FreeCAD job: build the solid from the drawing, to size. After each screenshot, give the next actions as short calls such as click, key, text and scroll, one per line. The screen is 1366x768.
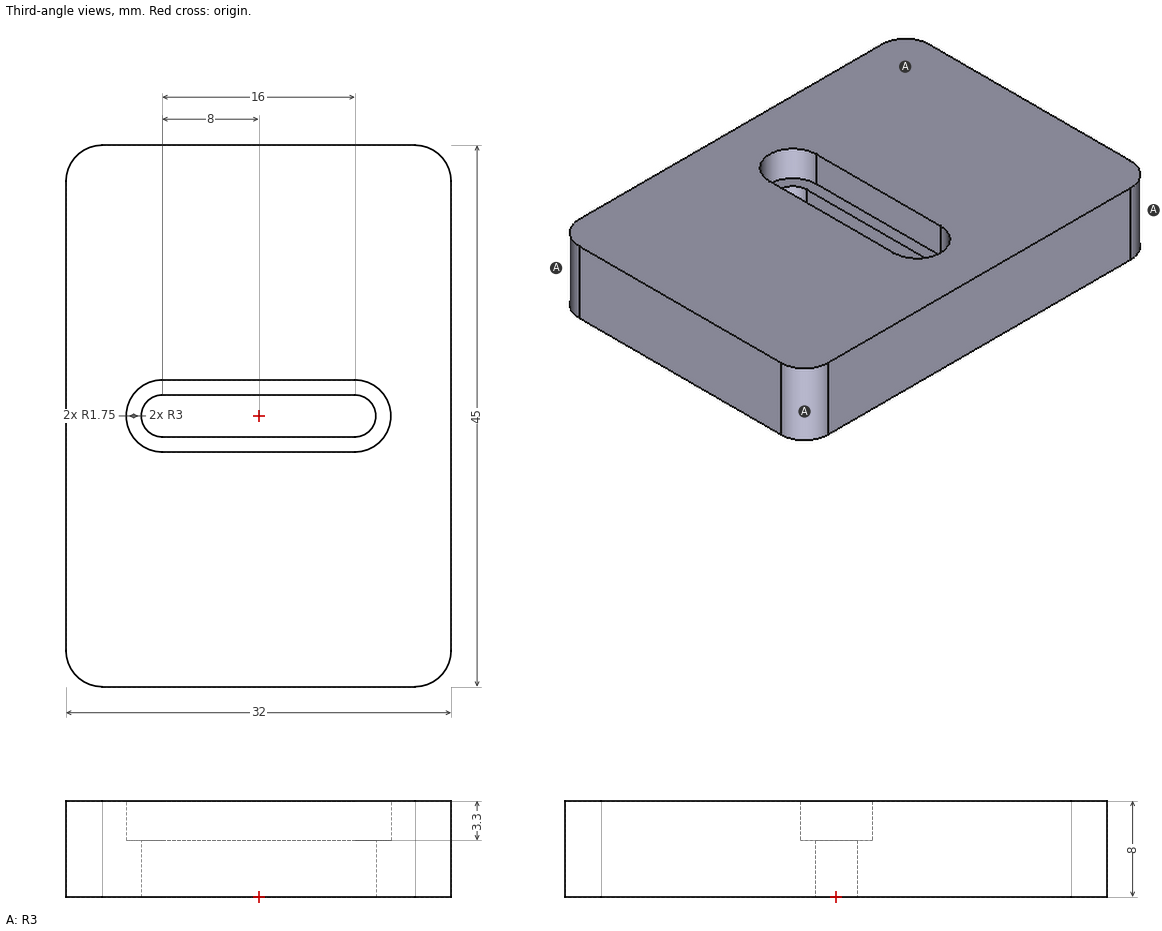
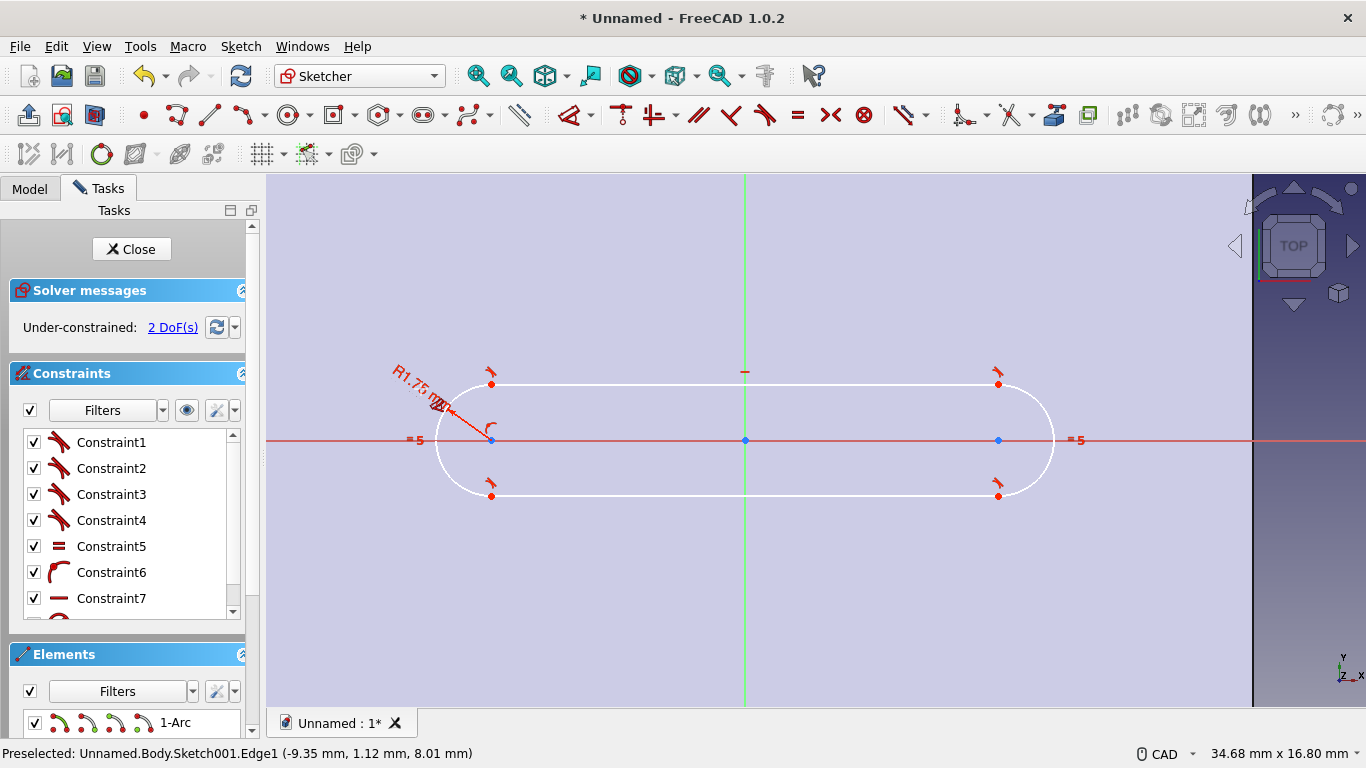
click(644, 385)
click(629, 351)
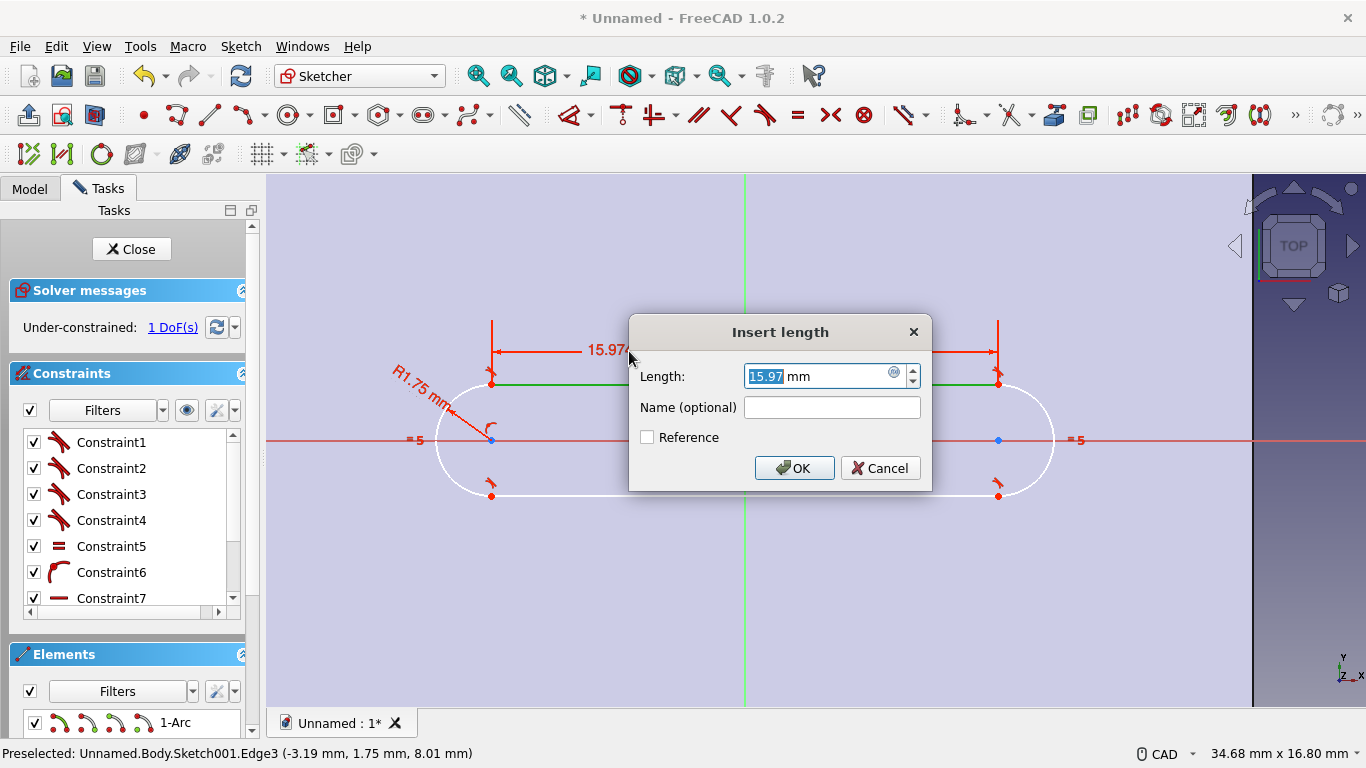
text(16)
key(Return)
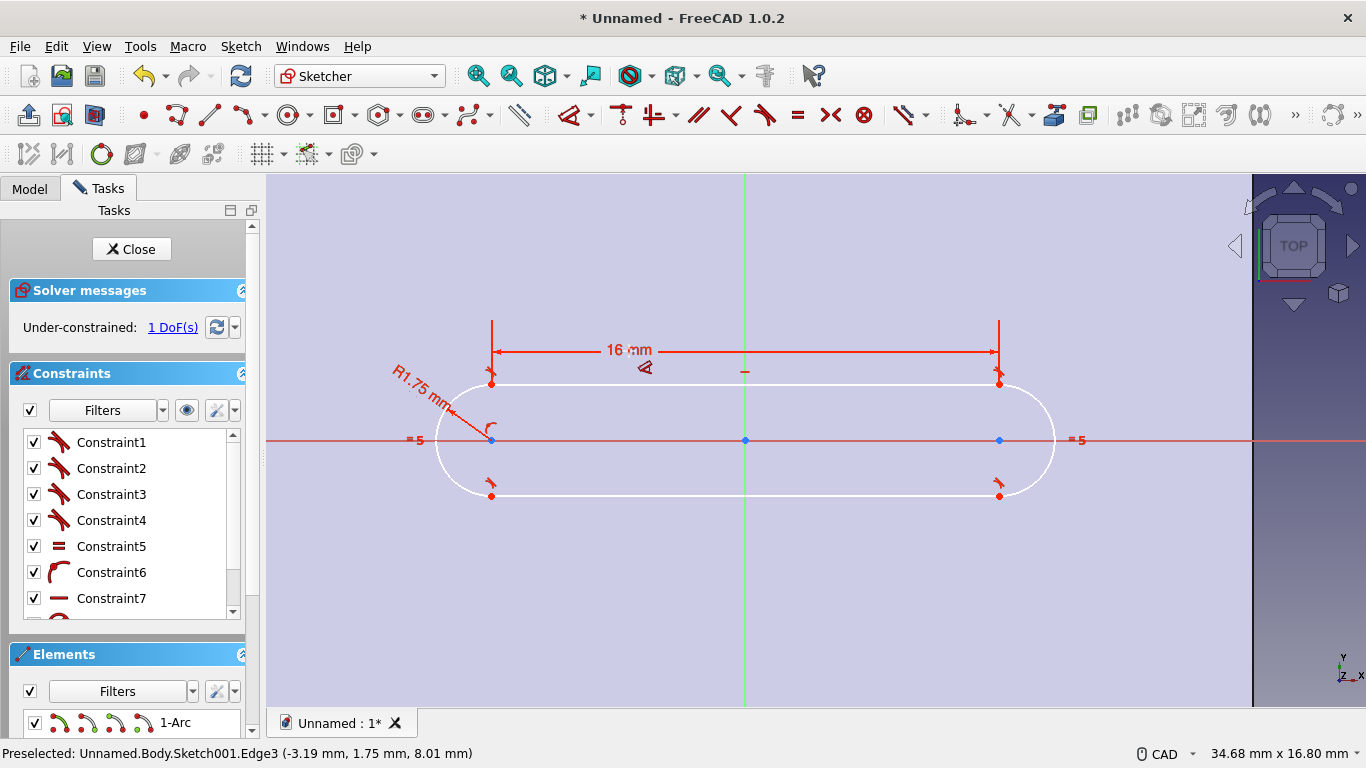
click(492, 385)
click(530, 351)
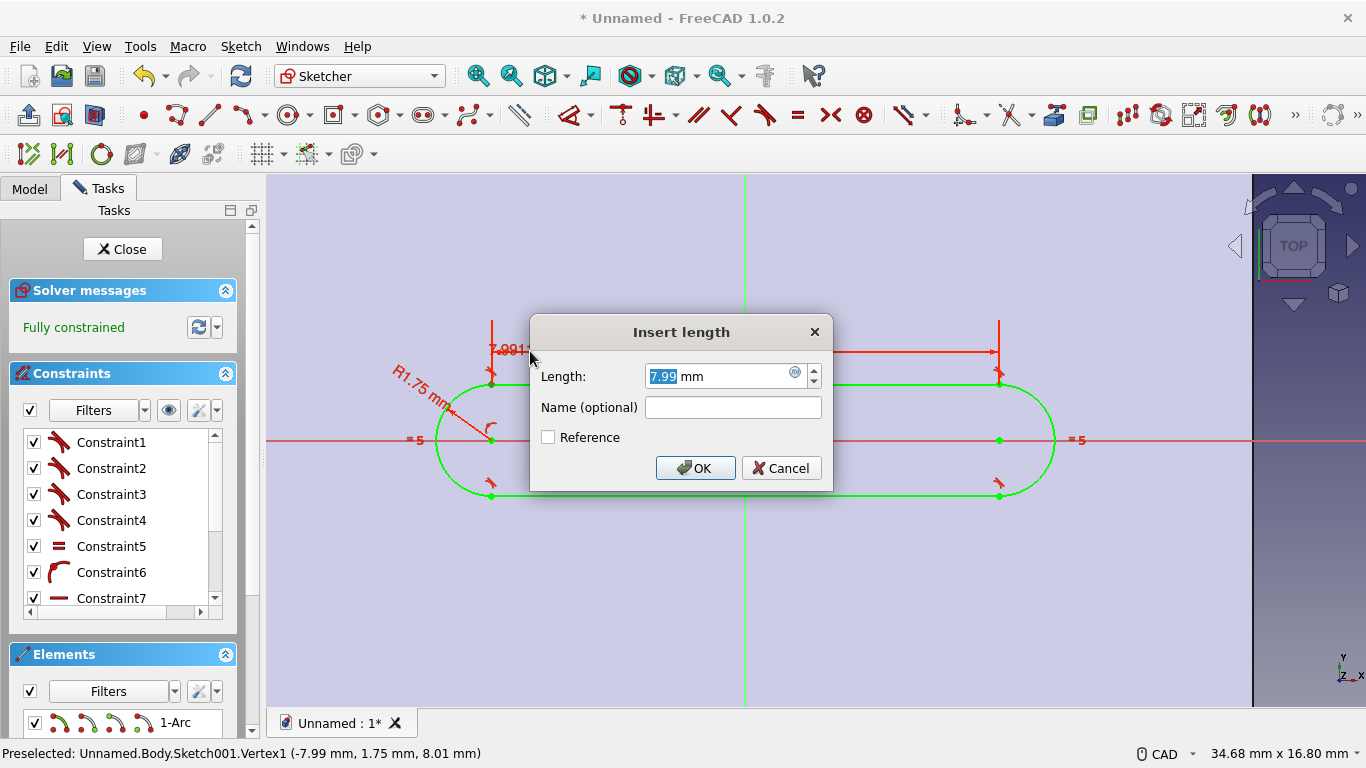
text(8)
key(Return)
key(Escape)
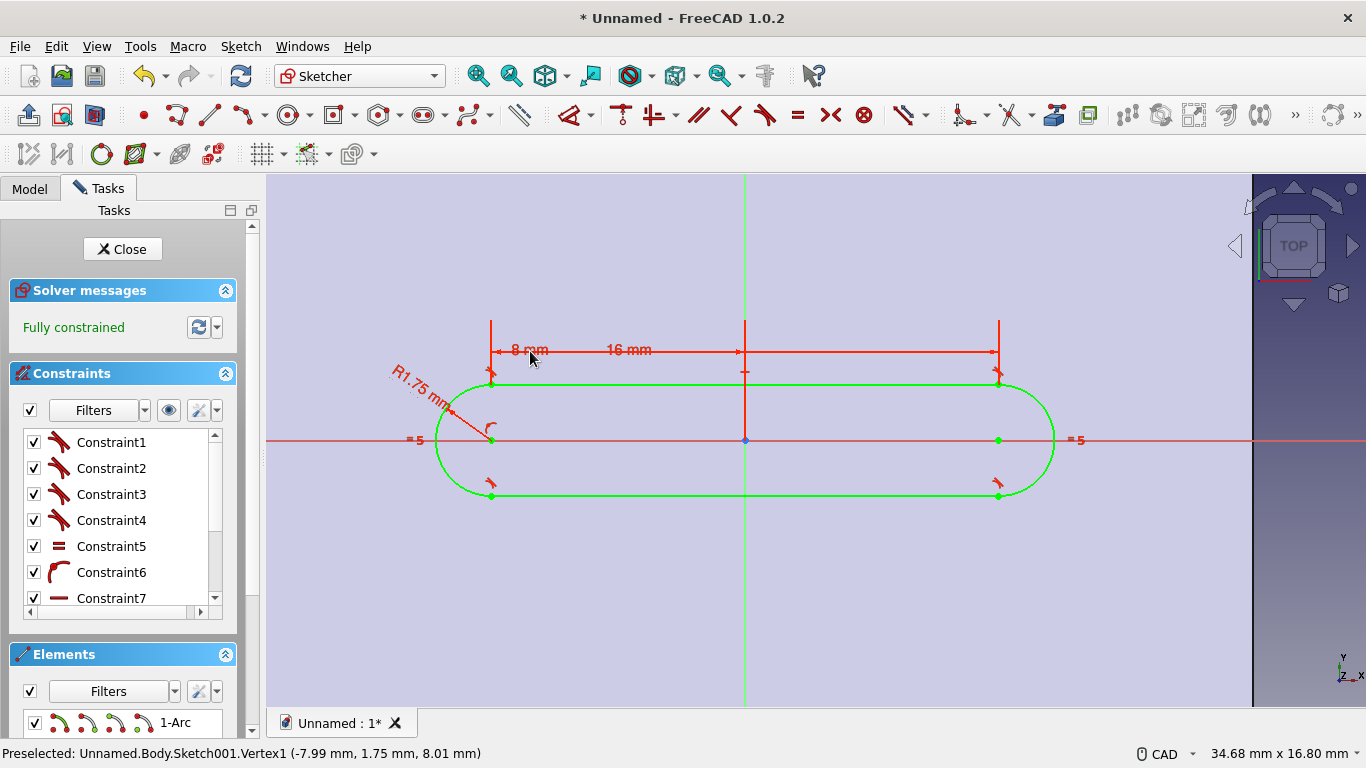
click(123, 249)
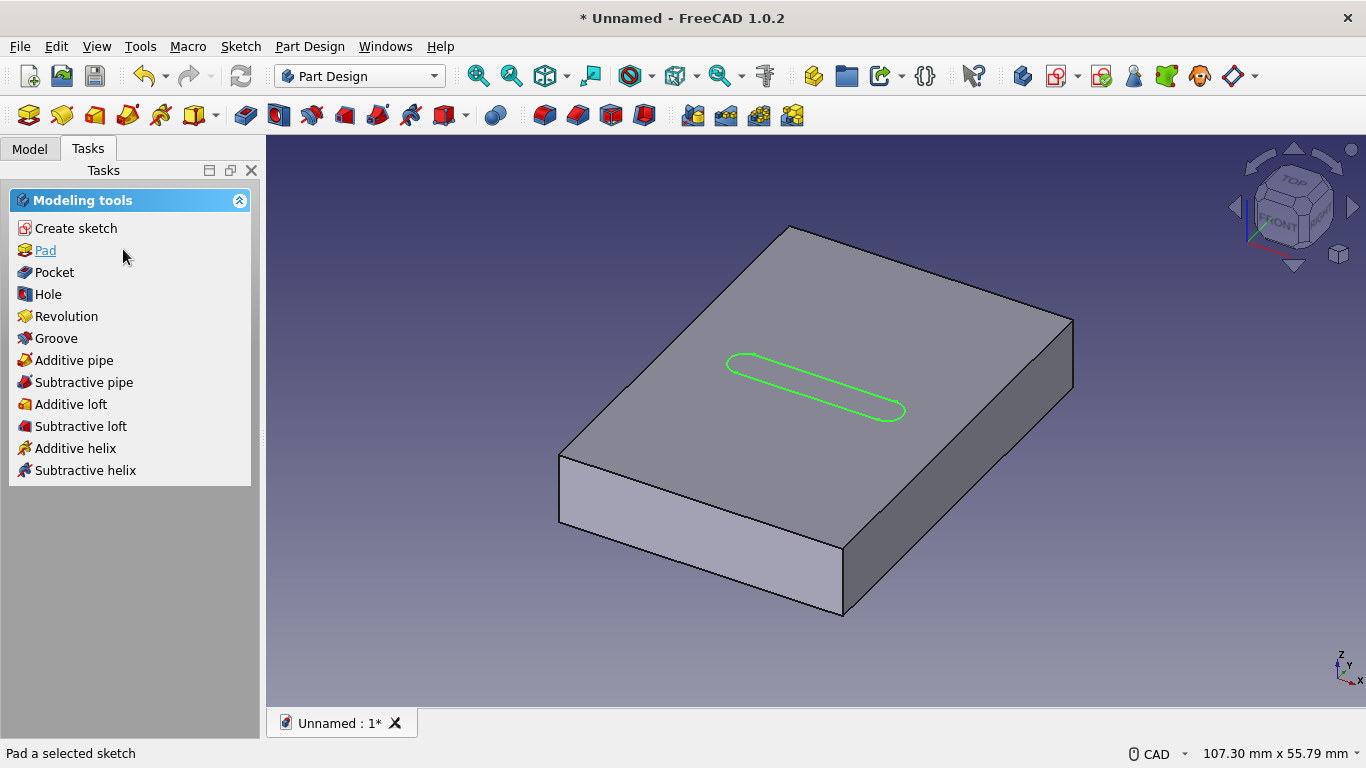
click(246, 116)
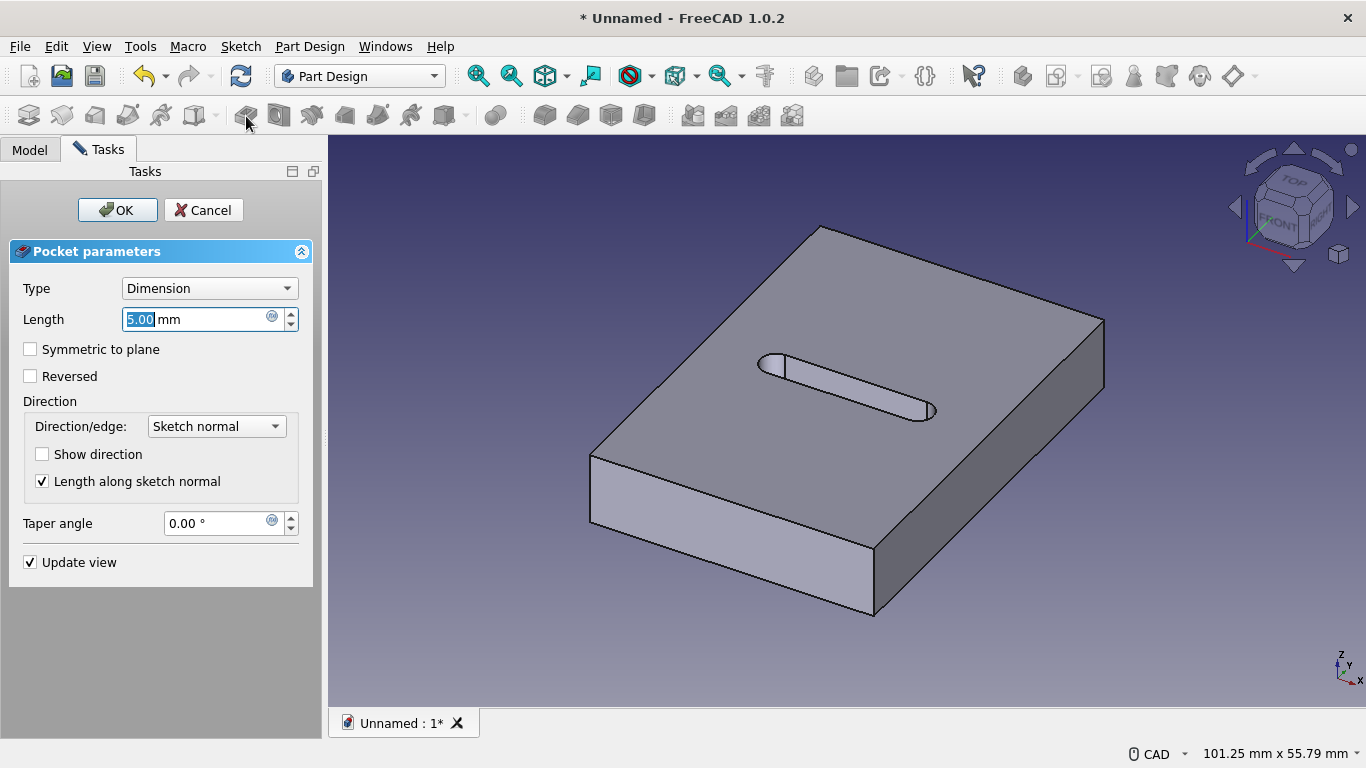
click(210, 288)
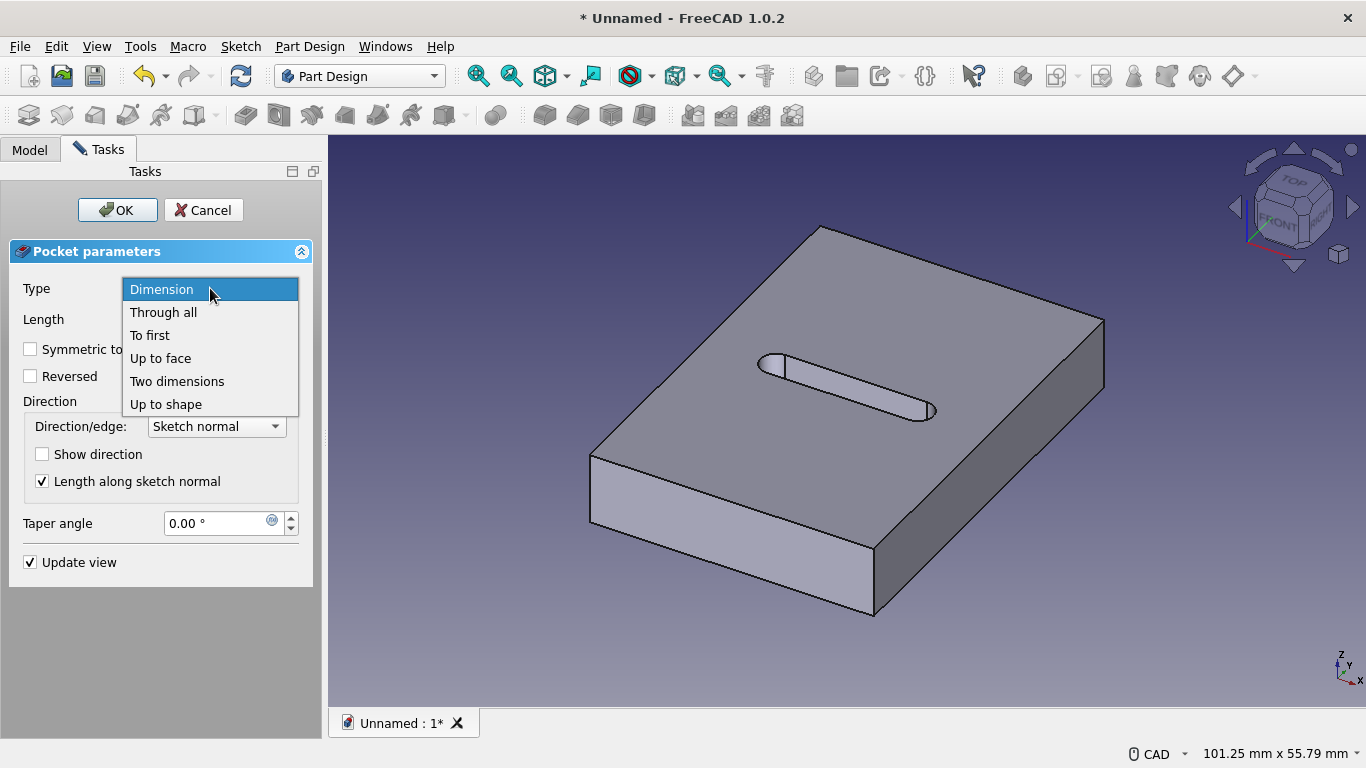
click(208, 312)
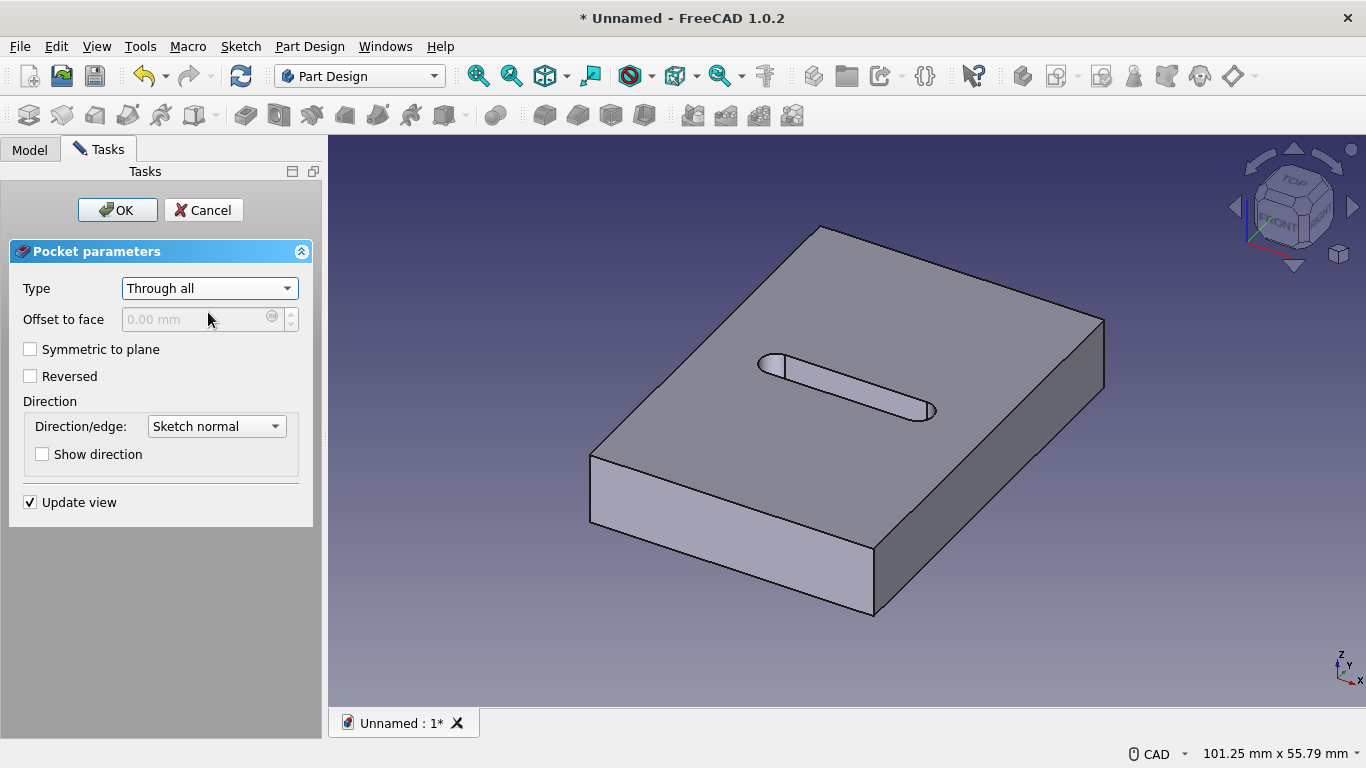
click(118, 210)